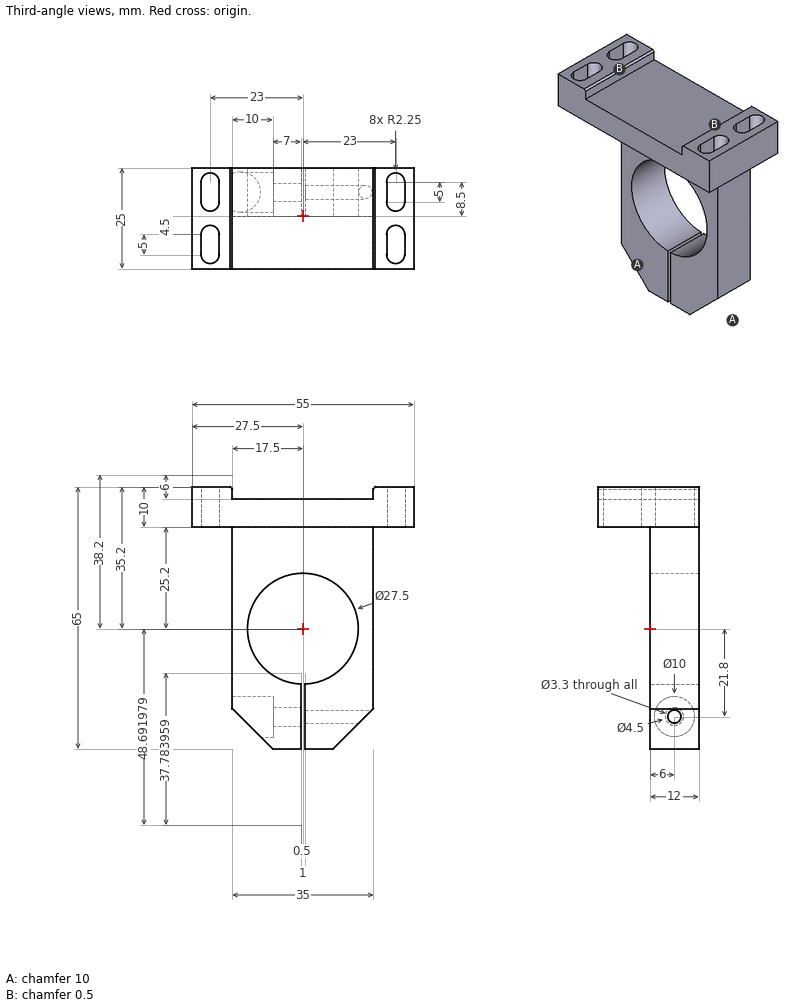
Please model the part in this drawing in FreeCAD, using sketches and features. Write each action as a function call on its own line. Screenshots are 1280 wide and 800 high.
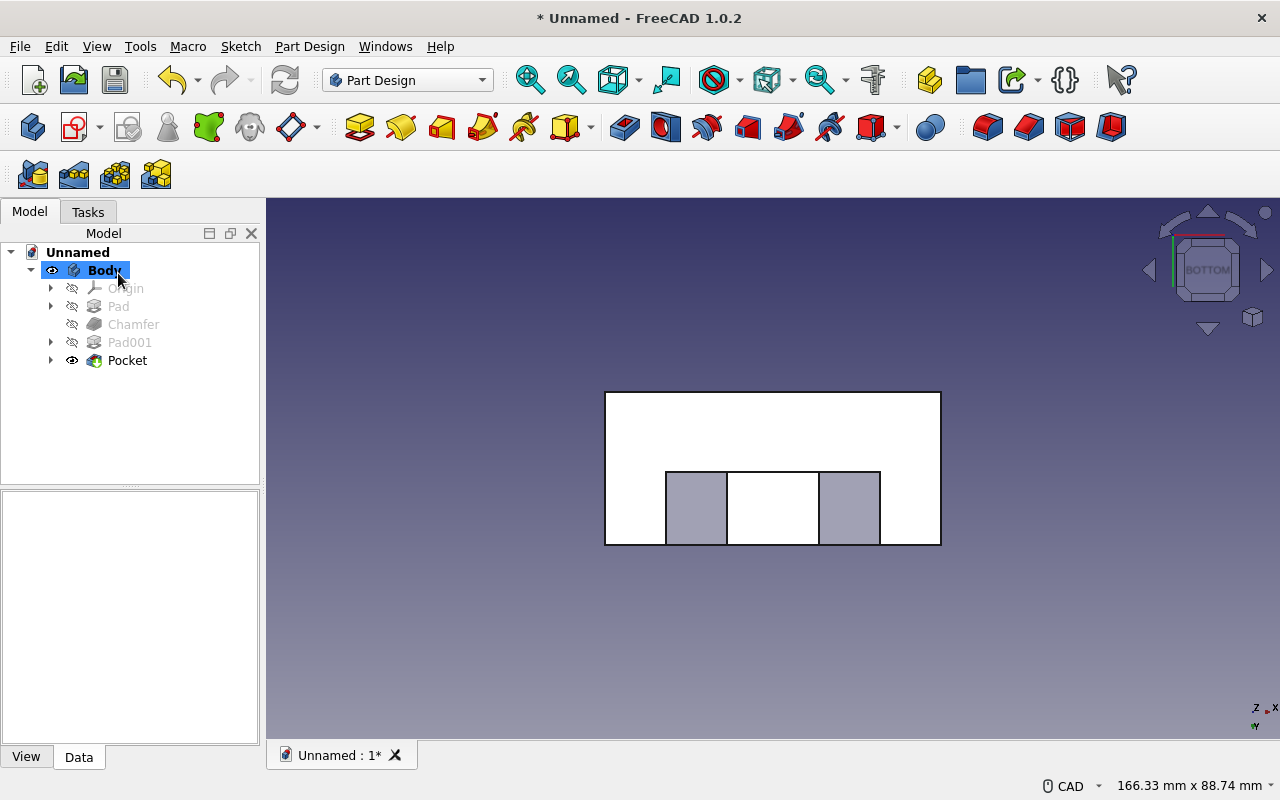
key(v)
key(f)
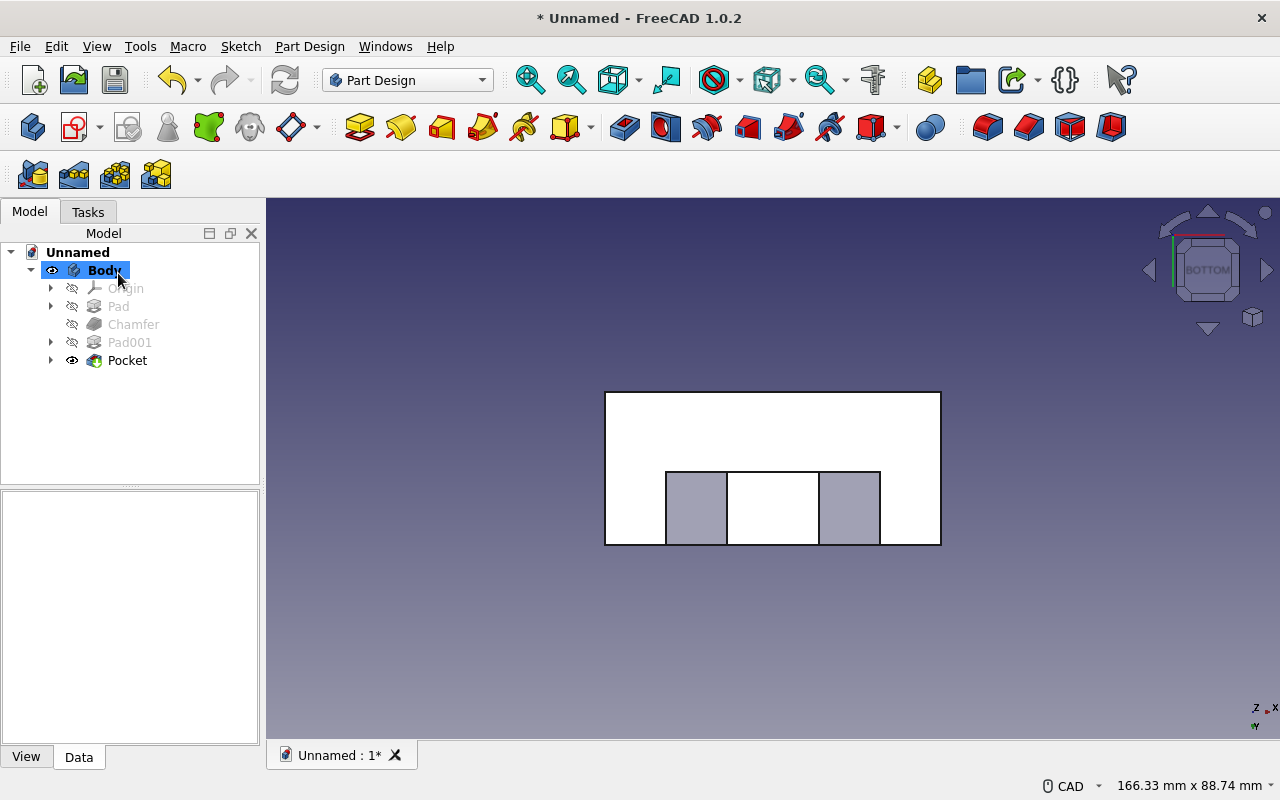
click(869, 424)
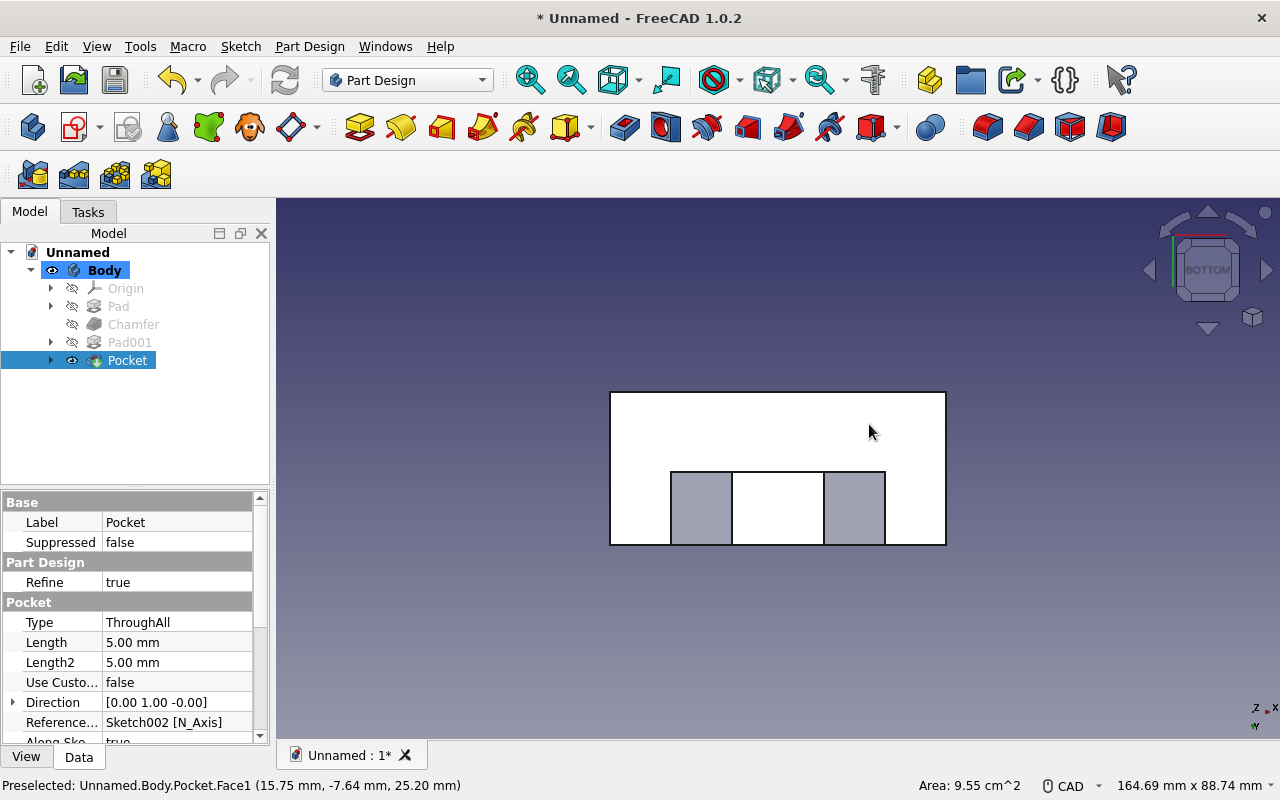
click(74, 128)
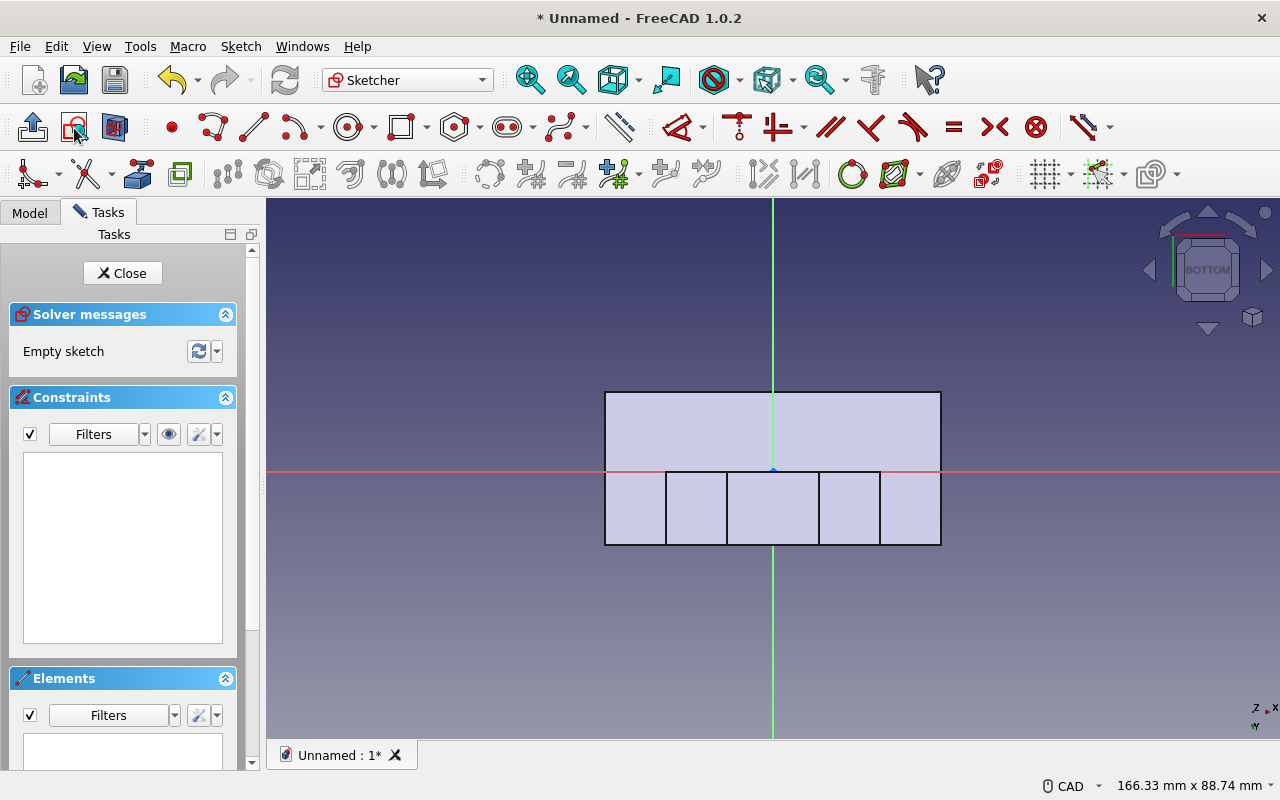
scroll(856, 468, up, 3)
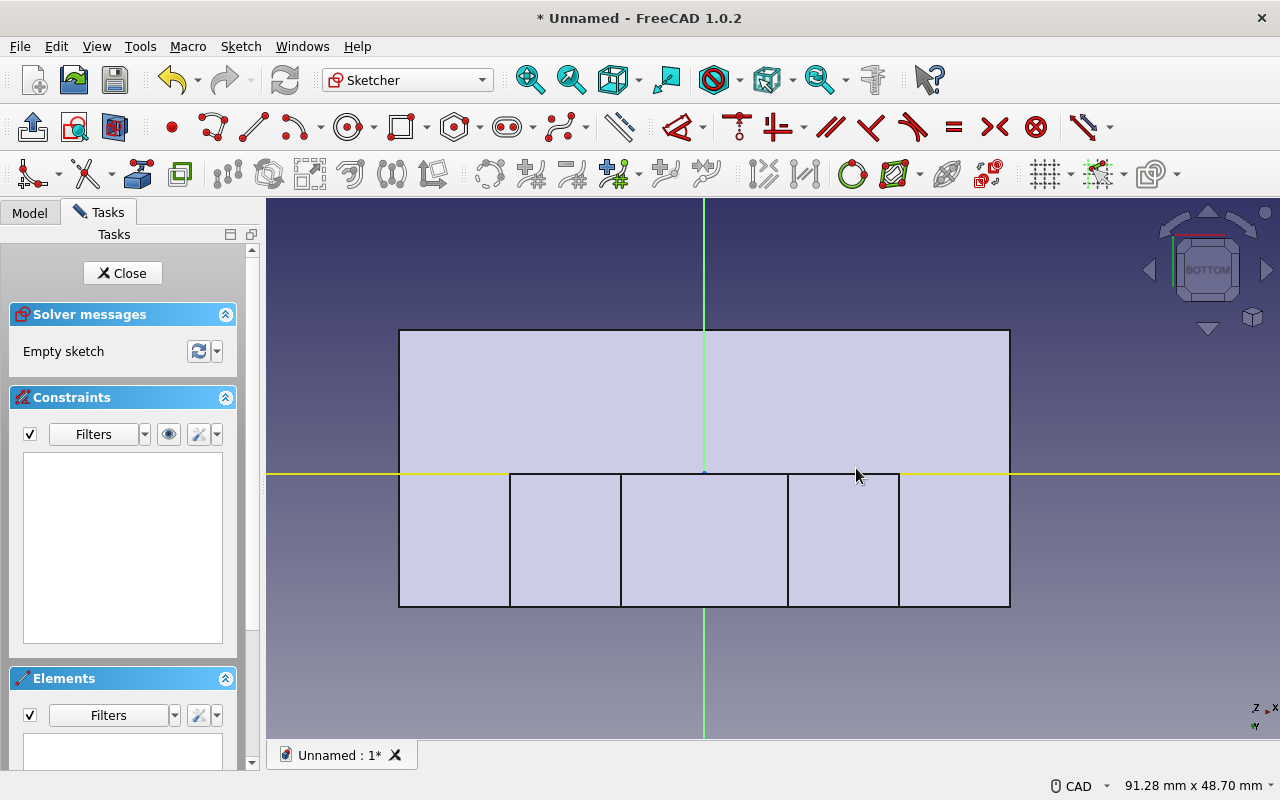
click(506, 128)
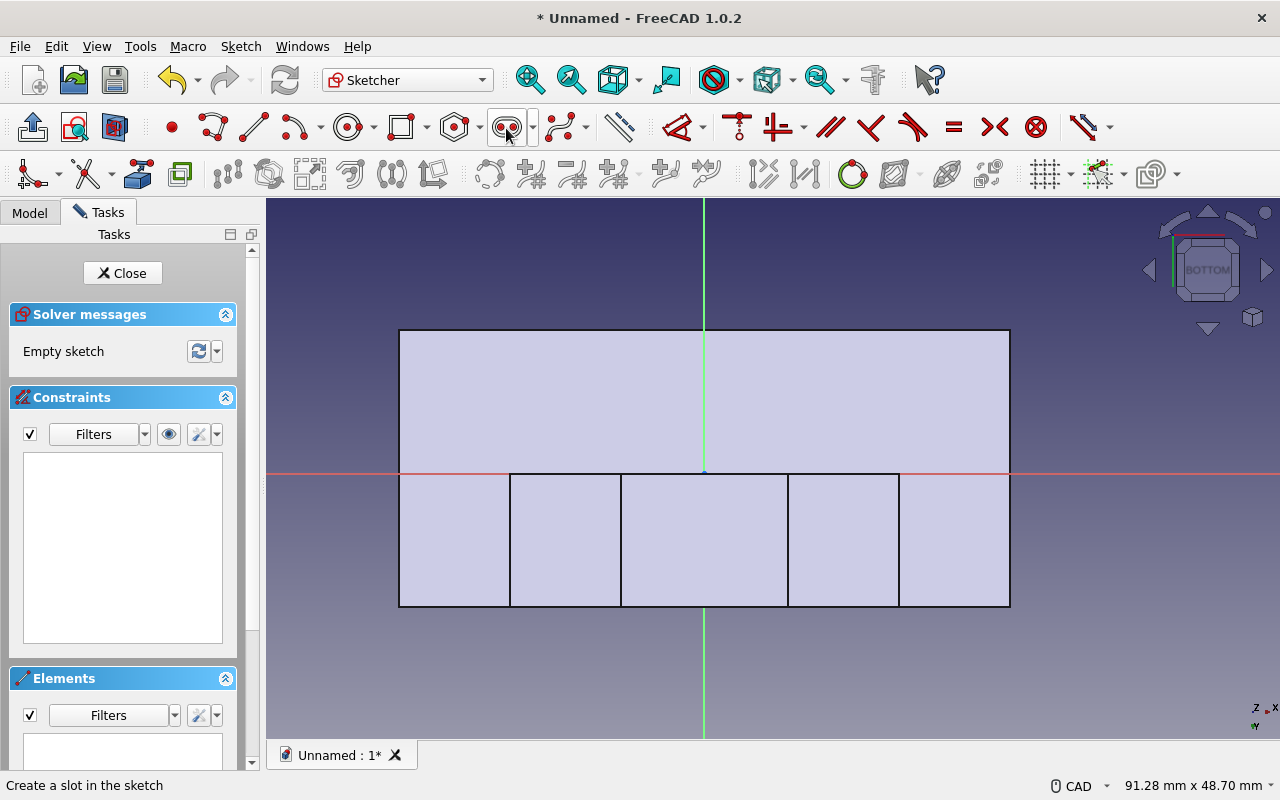
click(960, 568)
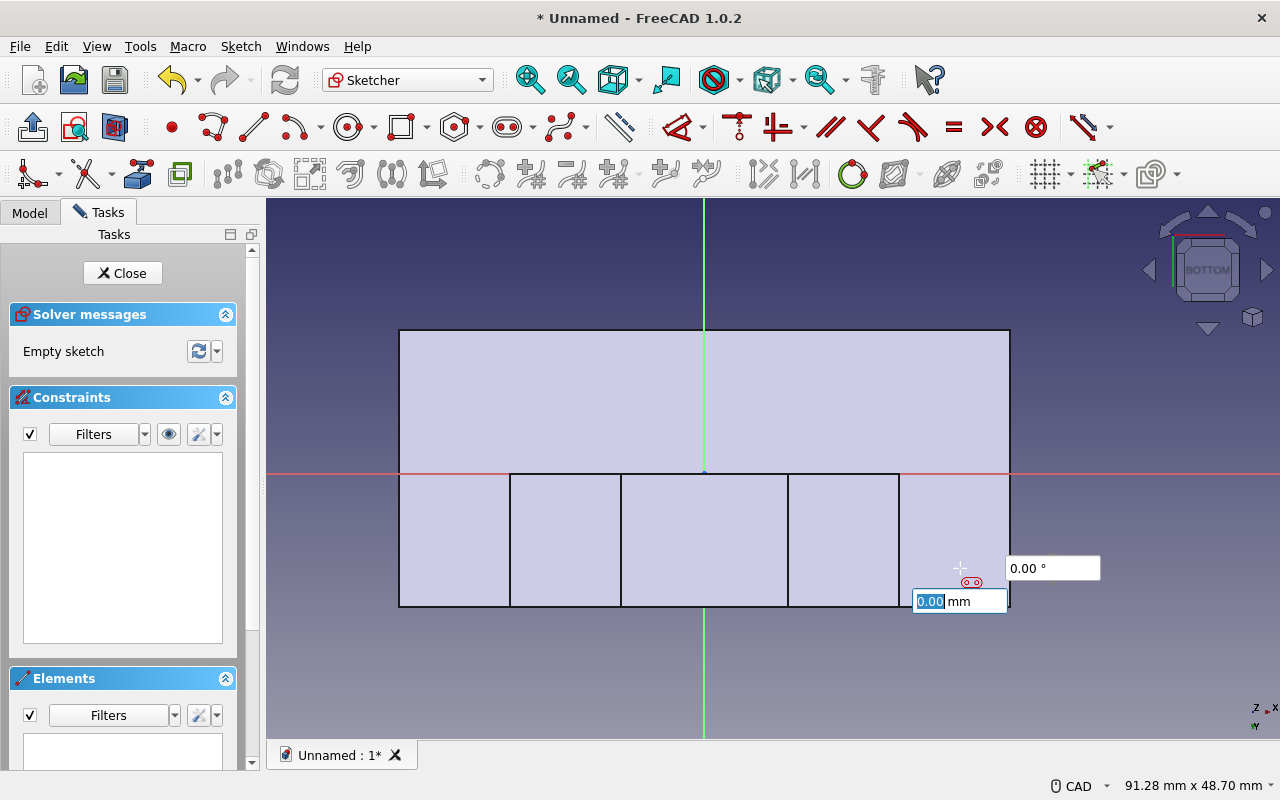
click(960, 513)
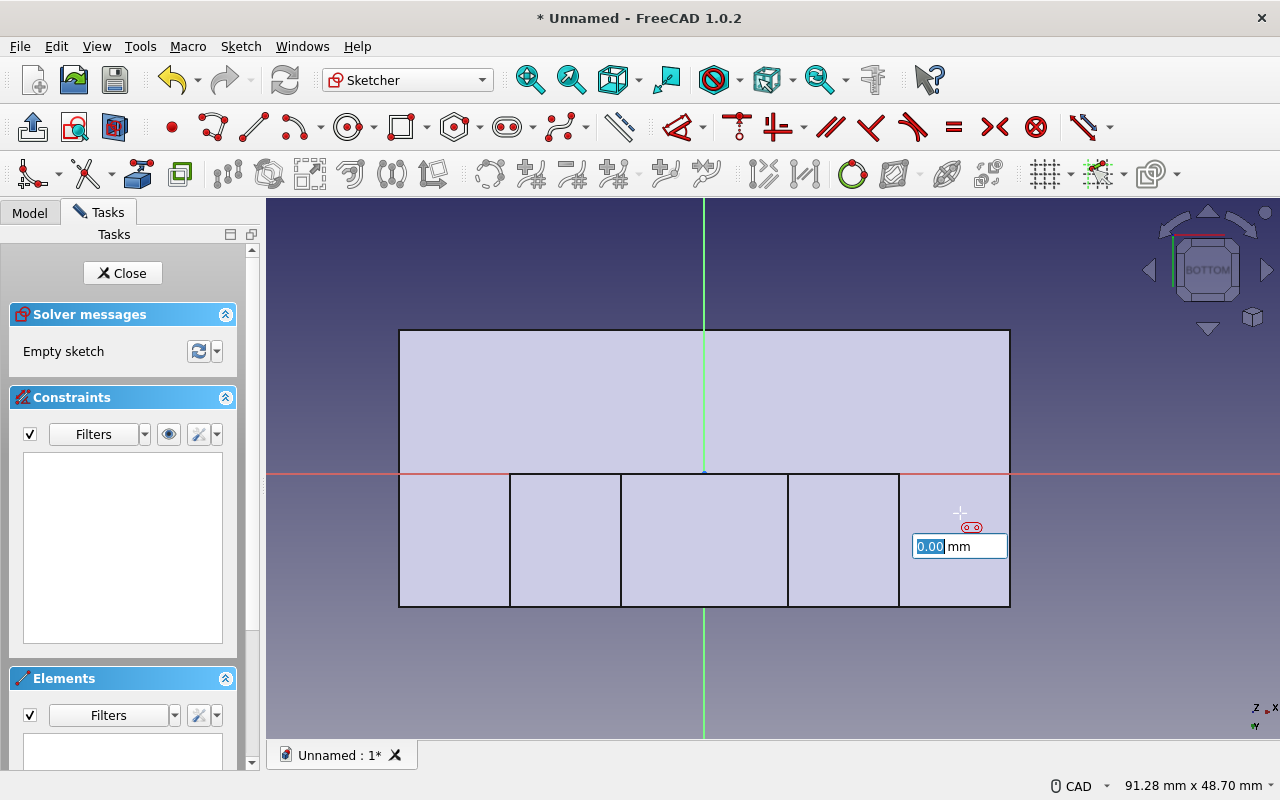
click(935, 541)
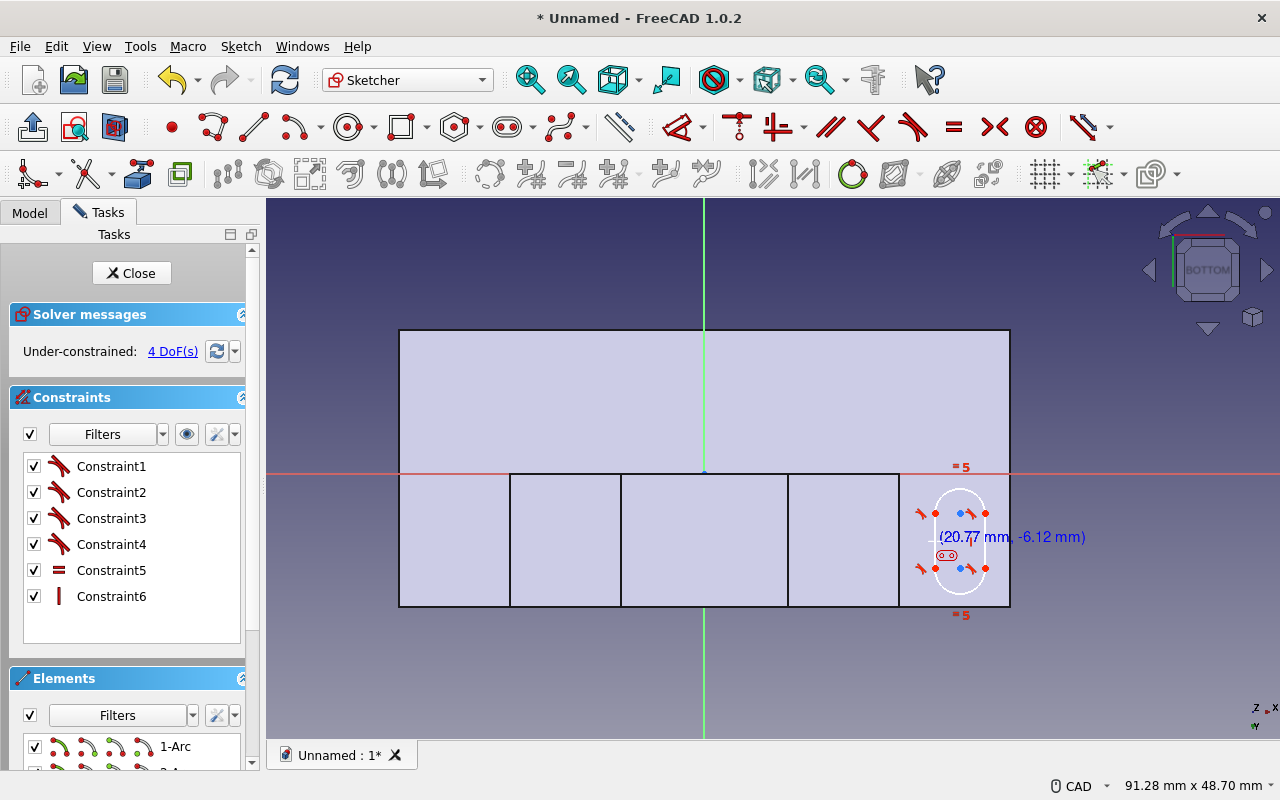
click(449, 568)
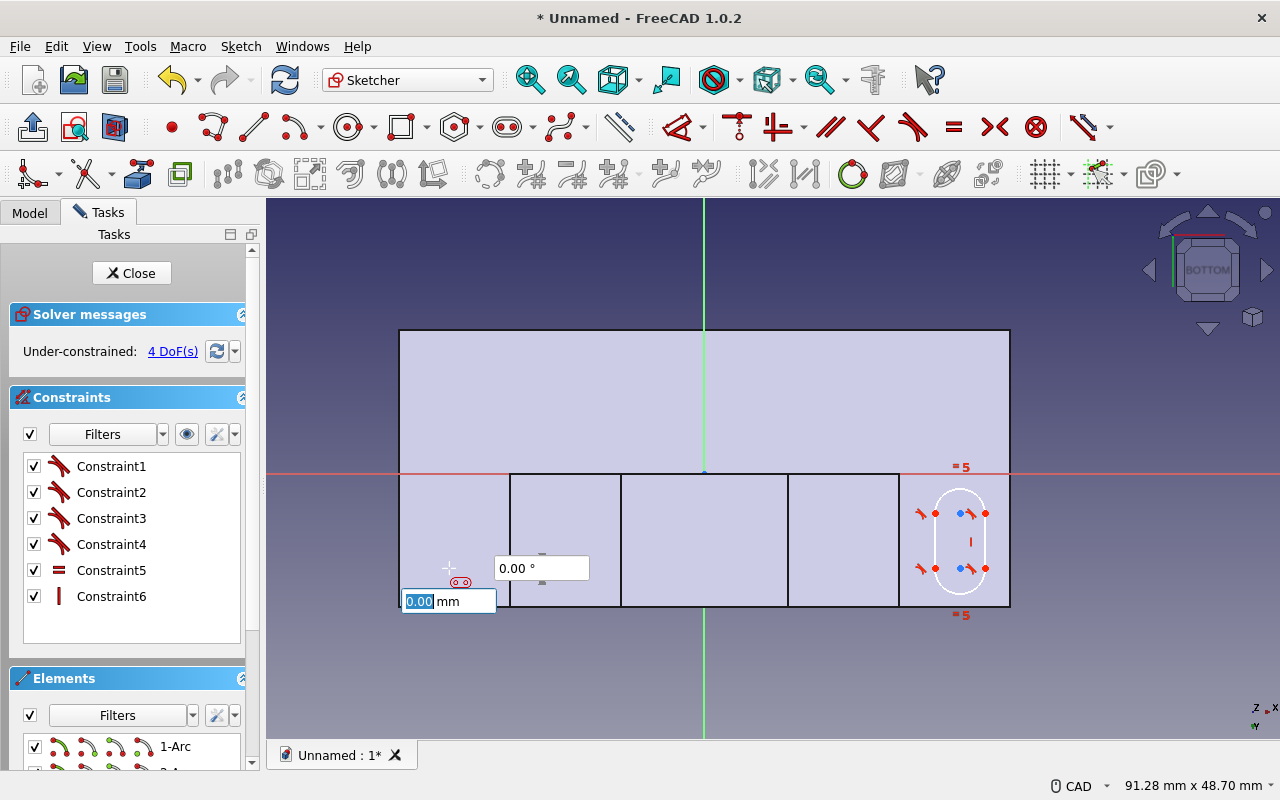
click(449, 513)